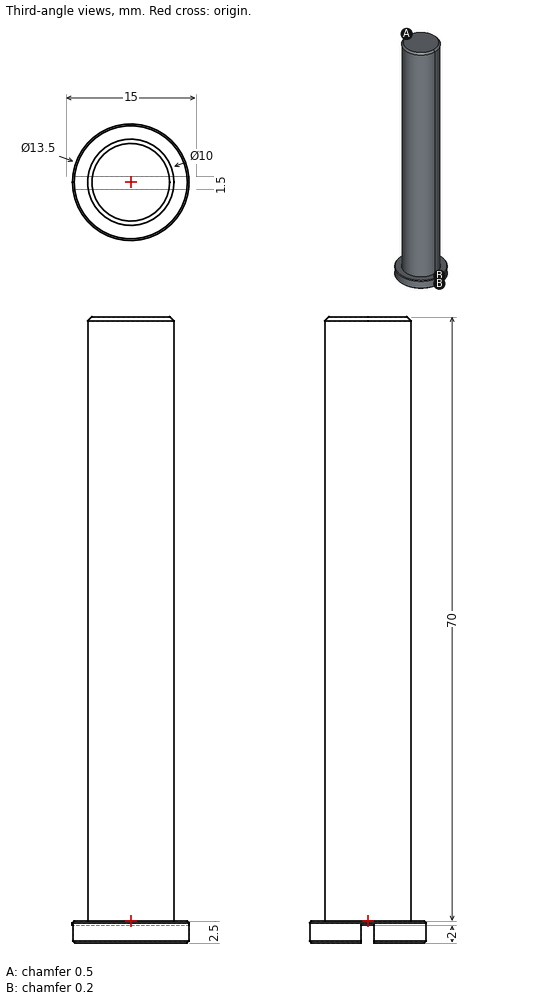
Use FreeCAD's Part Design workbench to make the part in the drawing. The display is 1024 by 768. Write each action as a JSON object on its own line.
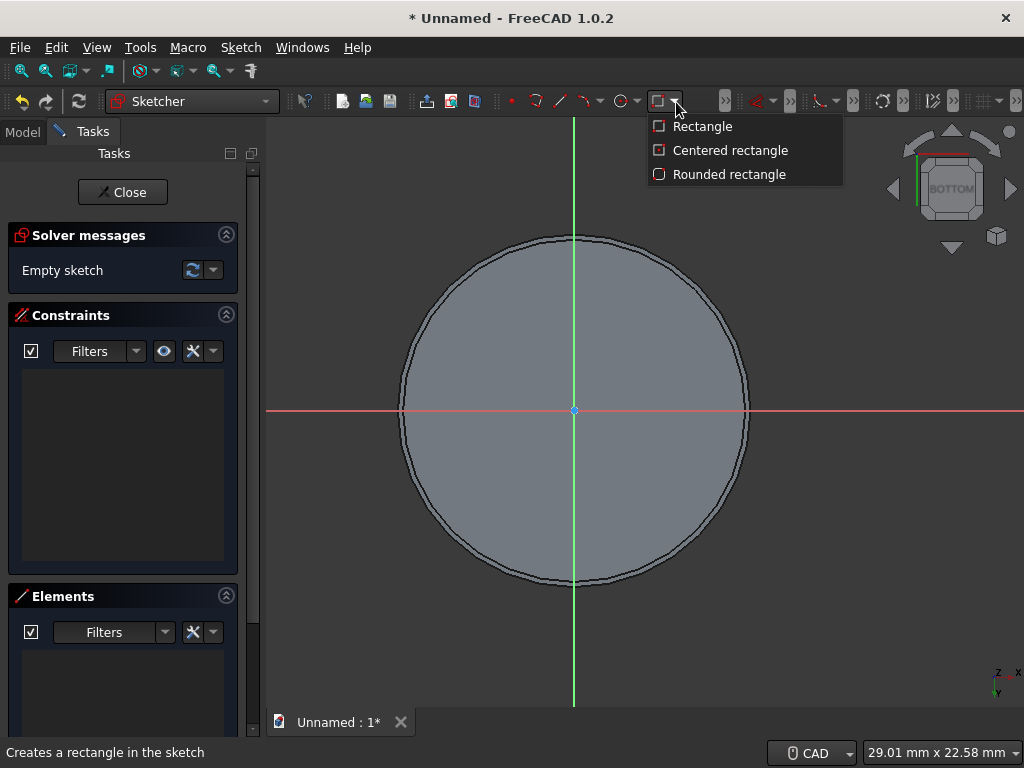
{"action": "left_click", "coordinate": [746, 150]}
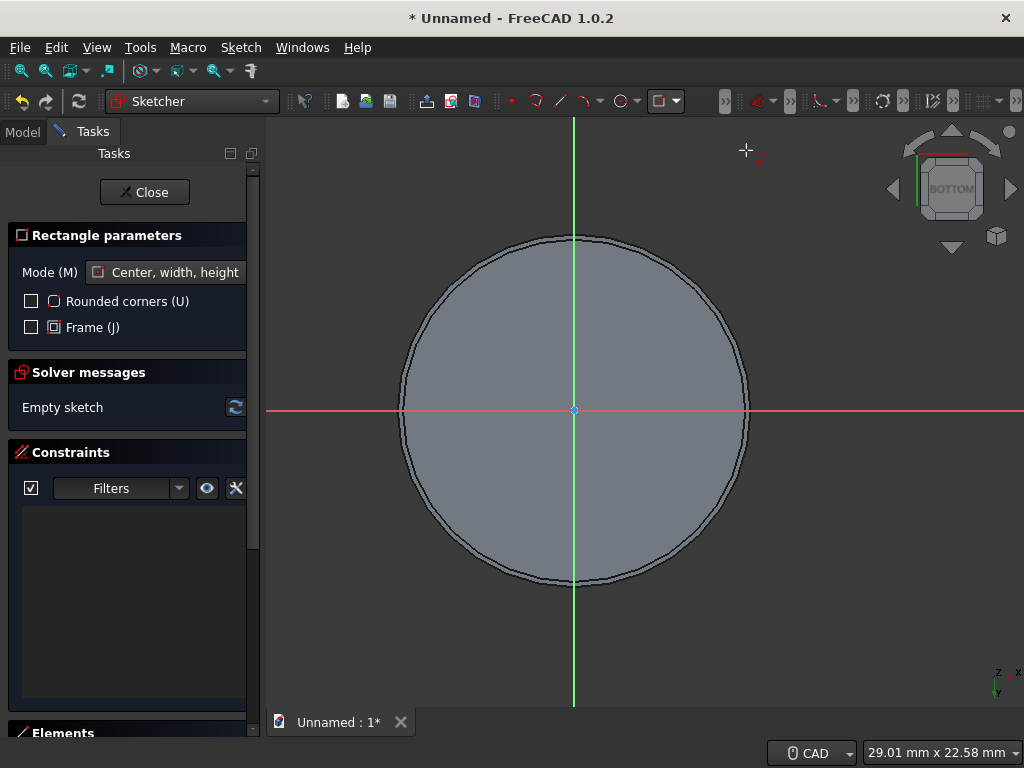
{"action": "left_click", "coordinate": [574, 411]}
{"action": "left_click", "coordinate": [770, 391]}
{"action": "key", "text": "Escape"}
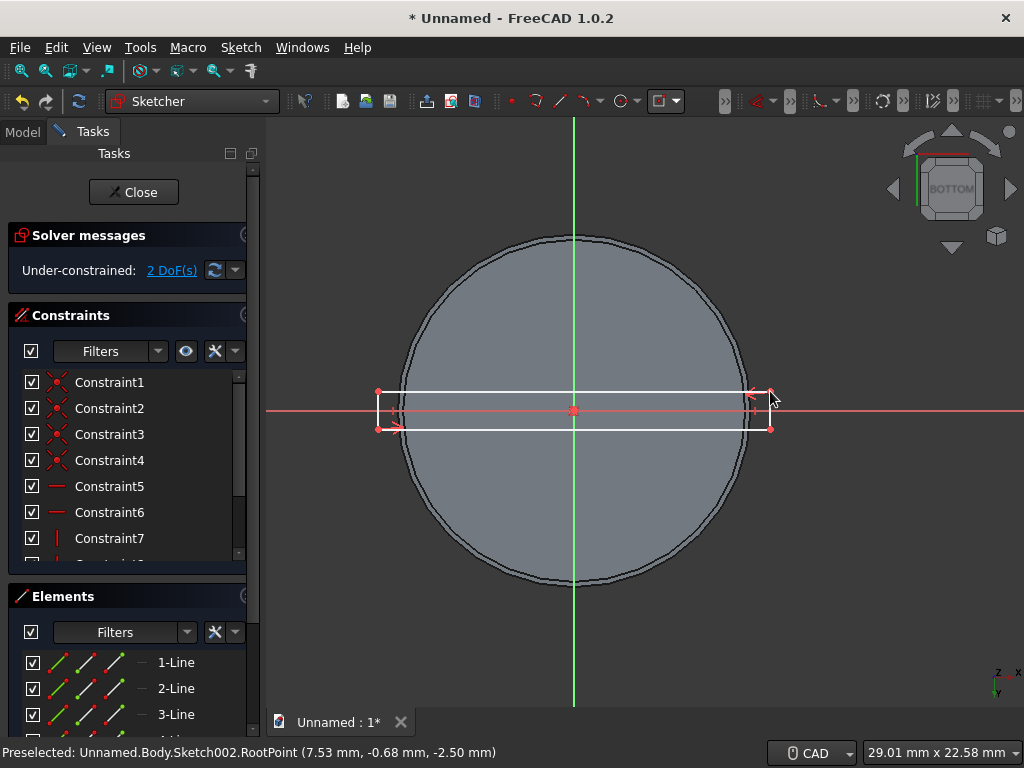
{"action": "left_click", "coordinate": [756, 102]}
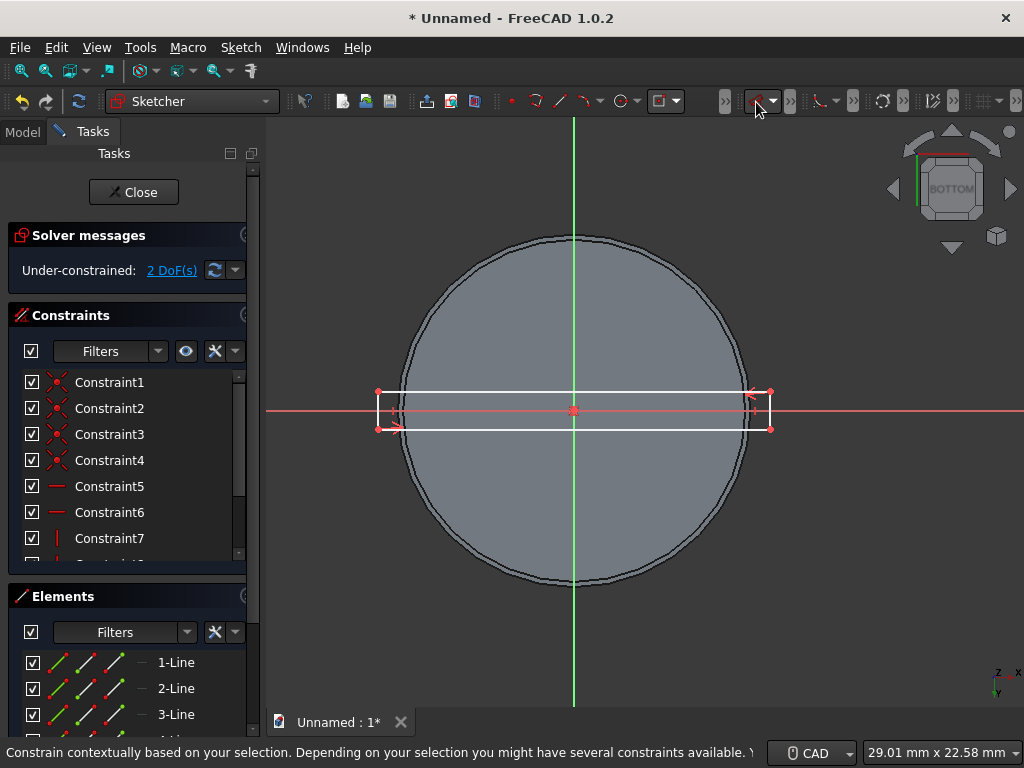
{"action": "left_click", "coordinate": [496, 430]}
{"action": "left_click", "coordinate": [484, 464]}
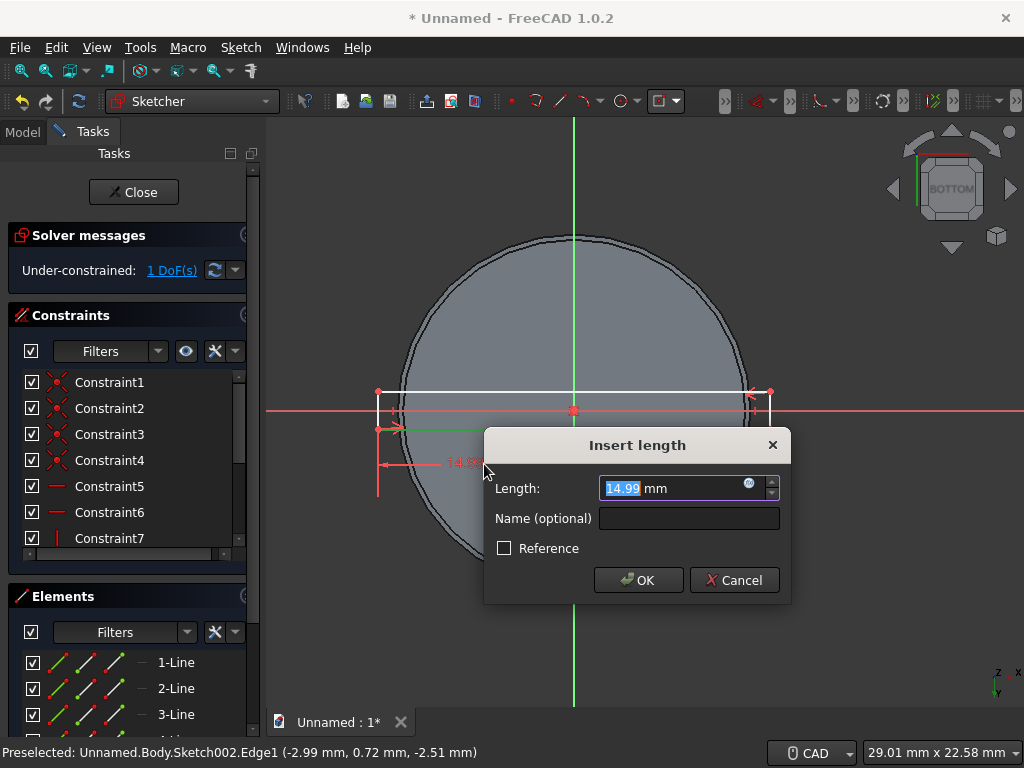
{"action": "type", "text": "15"}
{"action": "key", "text": "Return"}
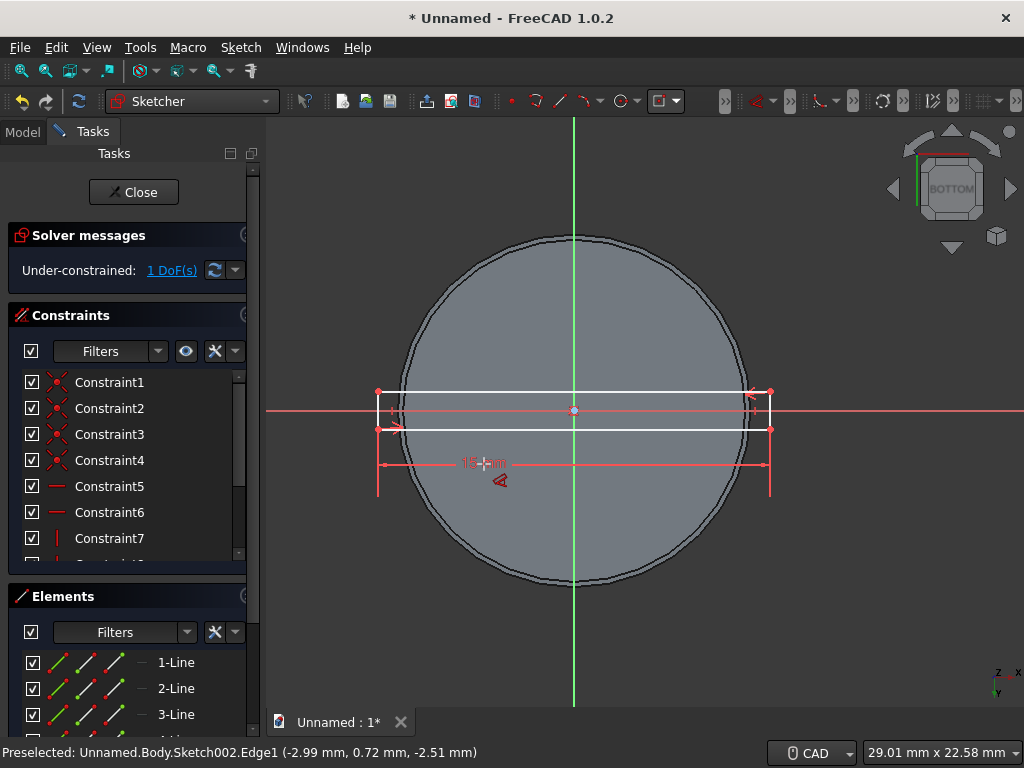
{"action": "left_click", "coordinate": [770, 415]}
{"action": "left_click", "coordinate": [804, 398]}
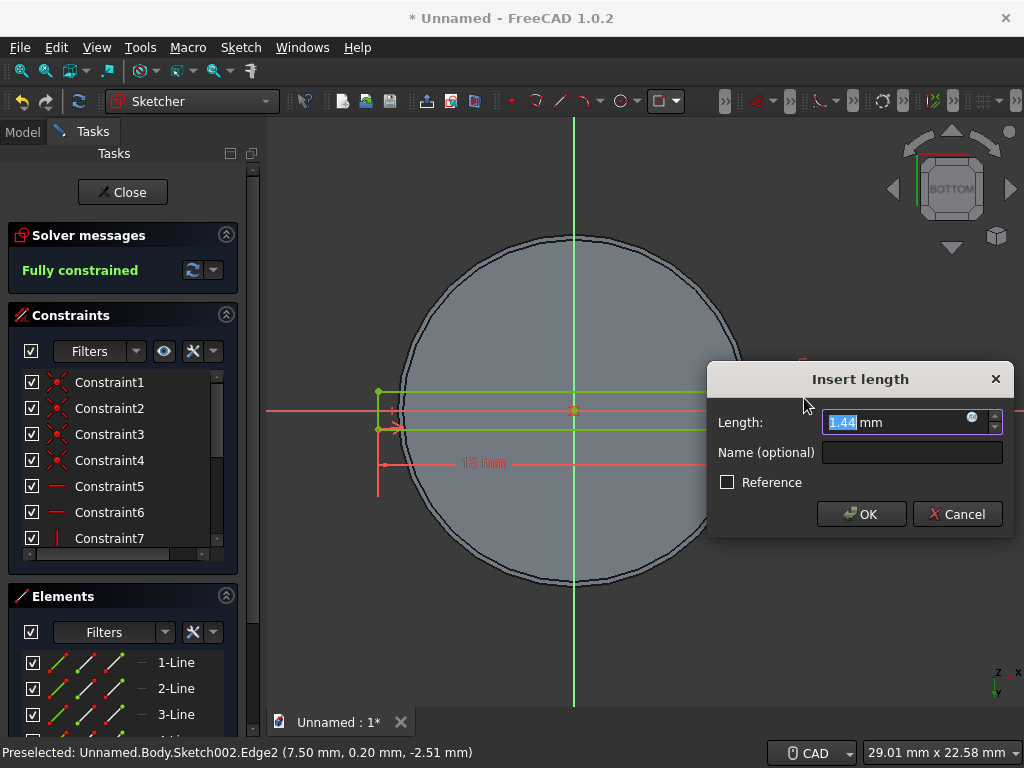
{"action": "type", "text": "1.5"}
{"action": "key", "text": "Return"}
{"action": "key", "text": "Escape"}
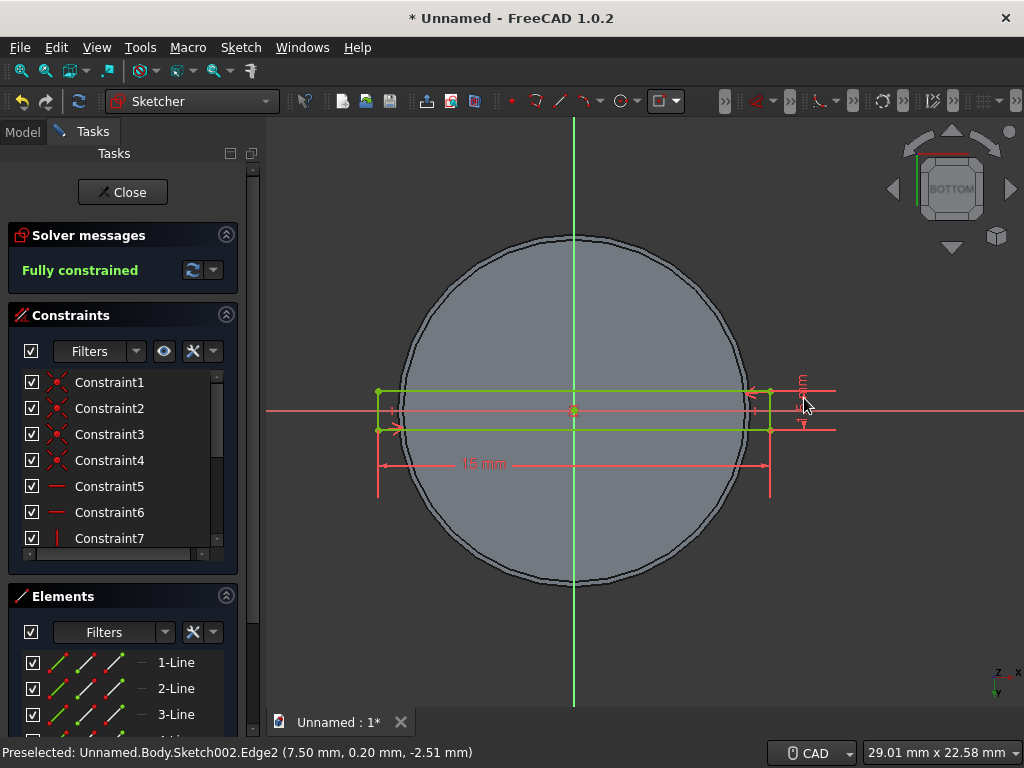
{"action": "left_click", "coordinate": [123, 192]}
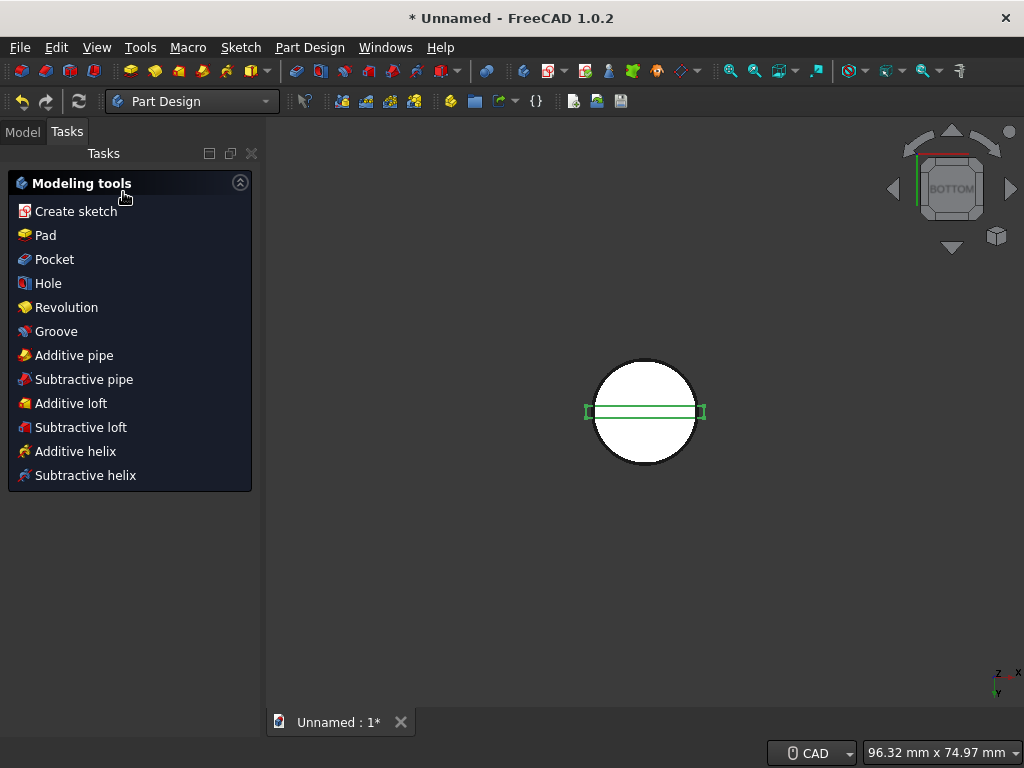
{"action": "left_click", "coordinate": [298, 72]}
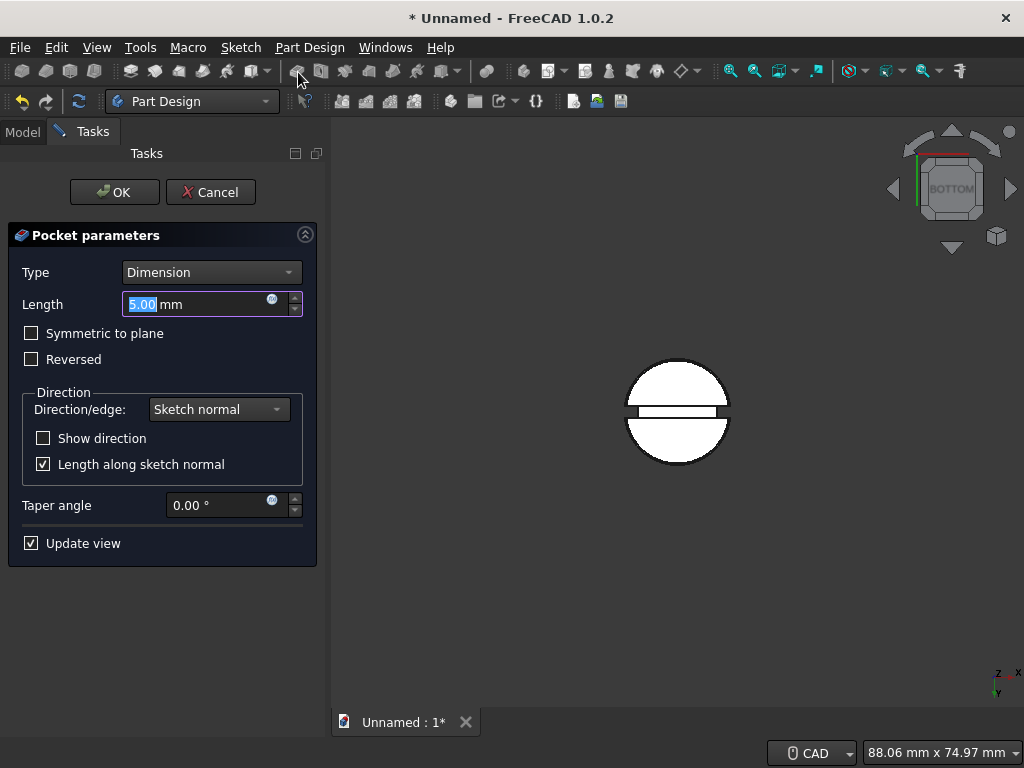
{"action": "type", "text": "2"}
{"action": "key", "text": "Tab"}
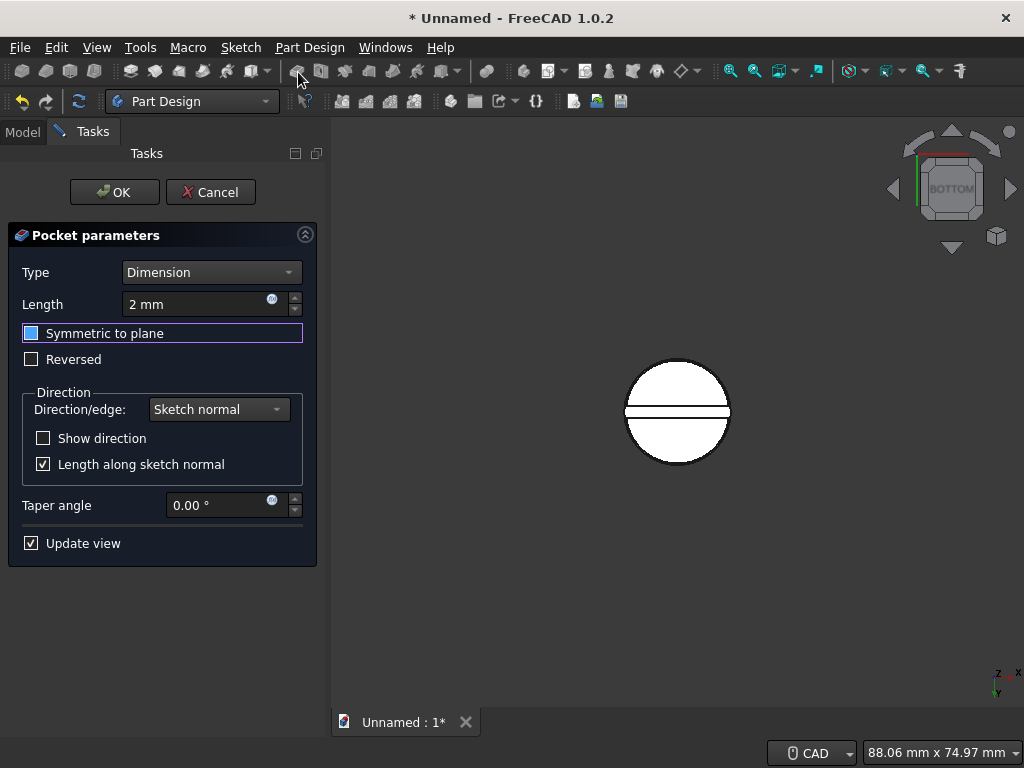
{"action": "left_click", "coordinate": [115, 192]}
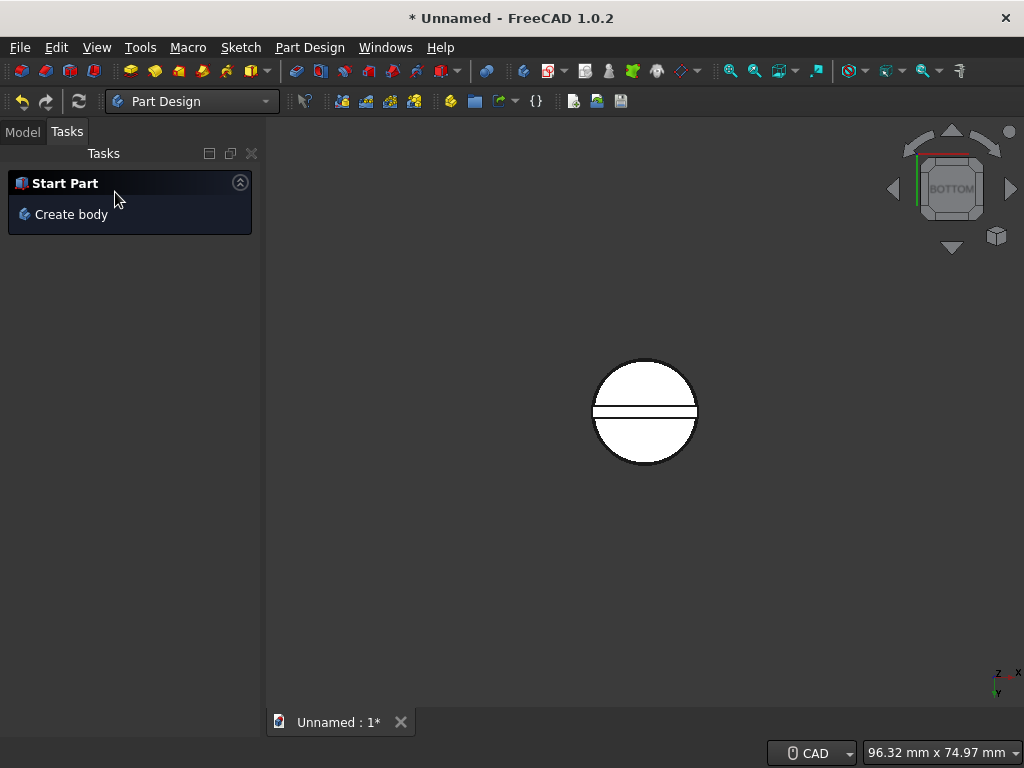
{"action": "key", "text": "0"}